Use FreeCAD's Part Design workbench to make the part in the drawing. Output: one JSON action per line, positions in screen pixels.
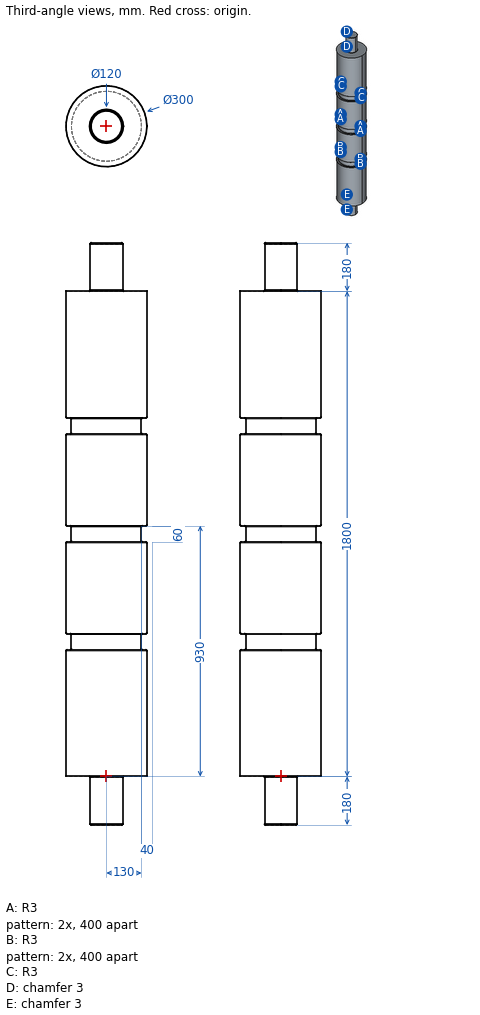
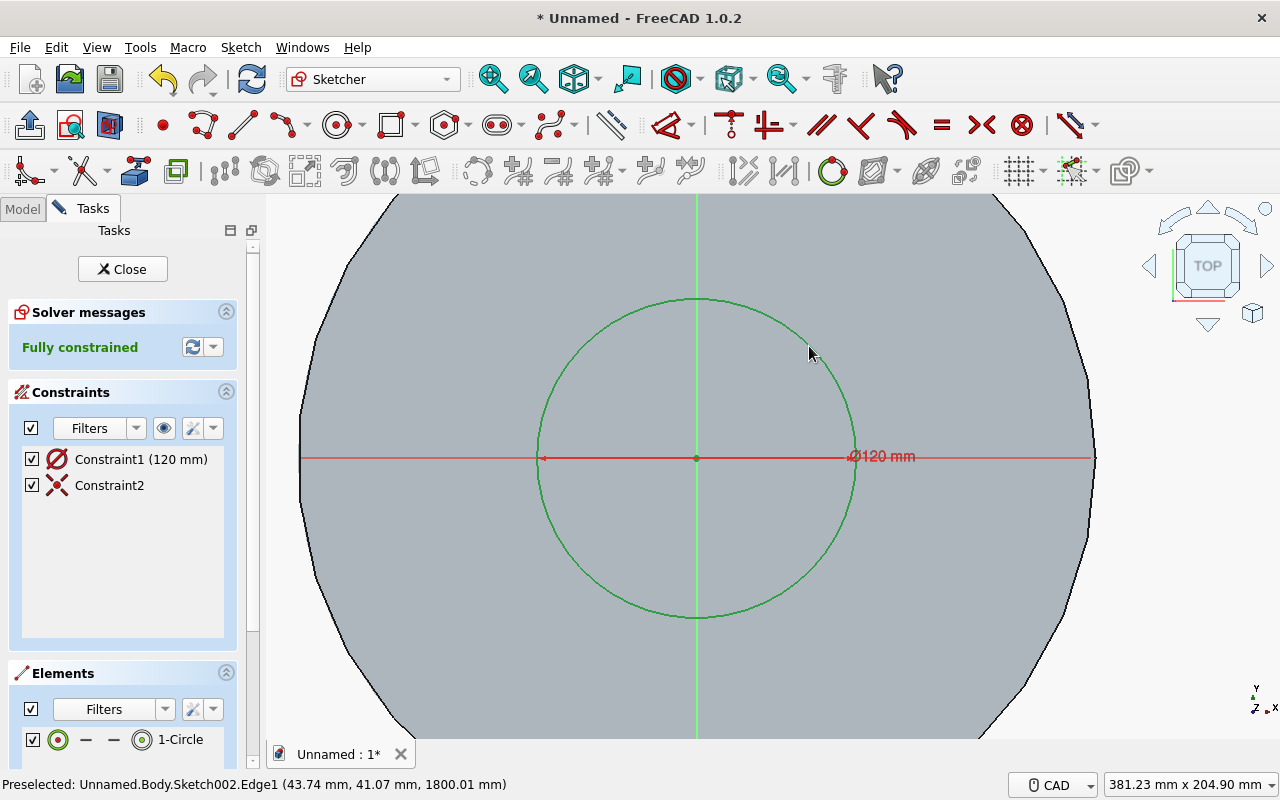
{"action": "left_click", "coordinate": [123, 269]}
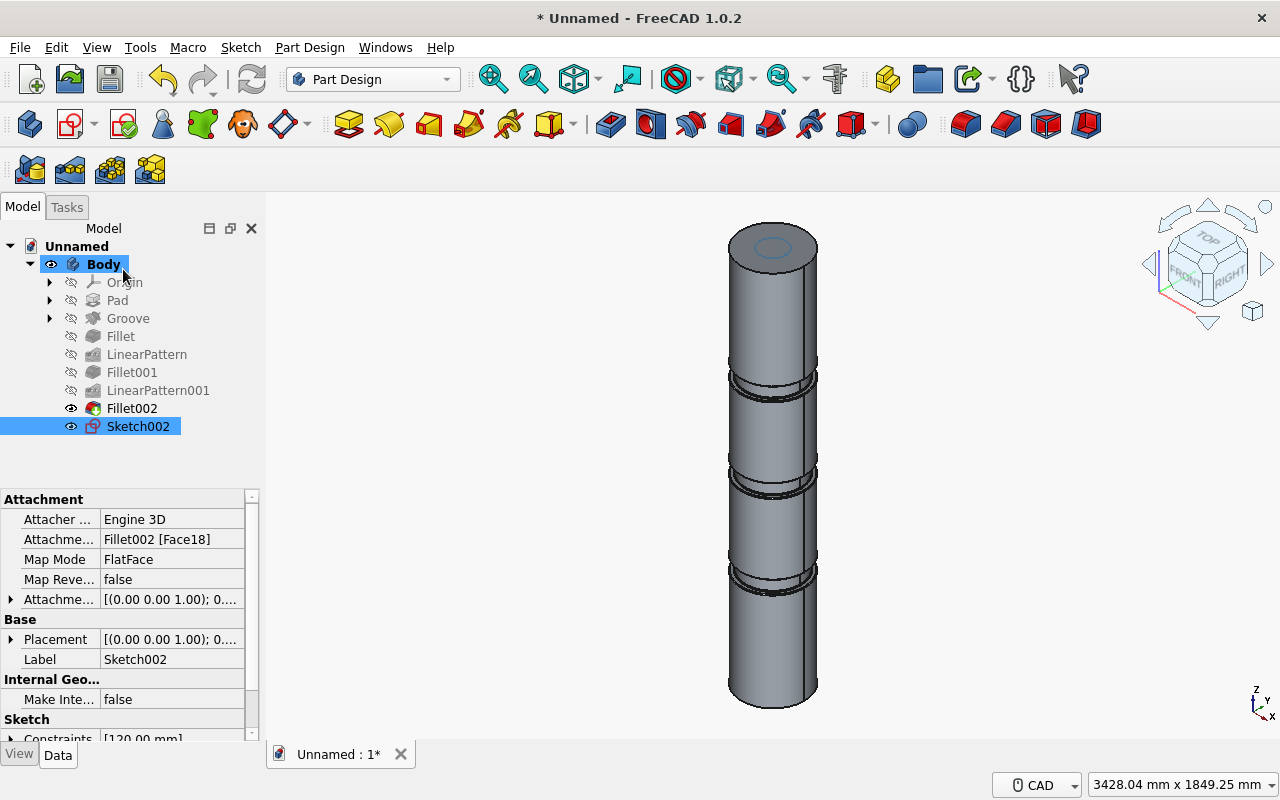
{"action": "left_click", "coordinate": [350, 124]}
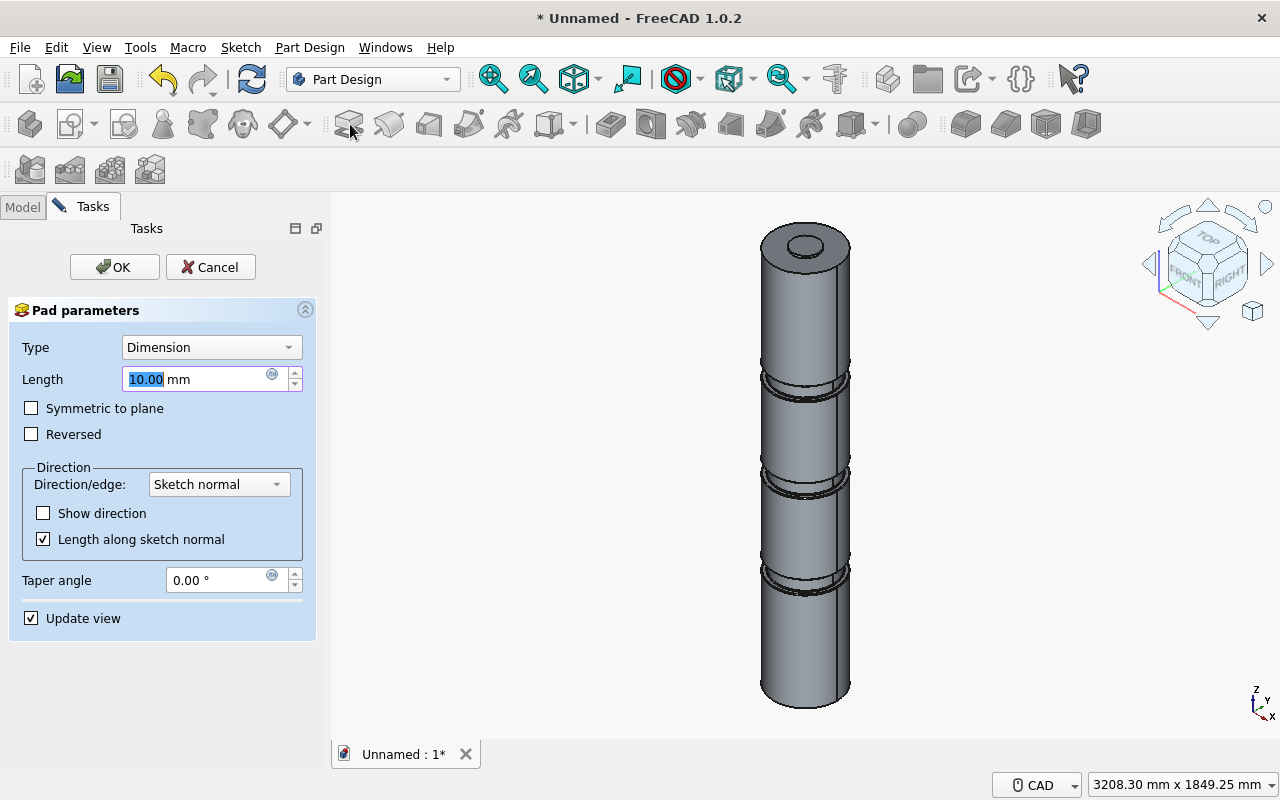
{"action": "type", "text": "180"}
{"action": "key", "text": "Tab"}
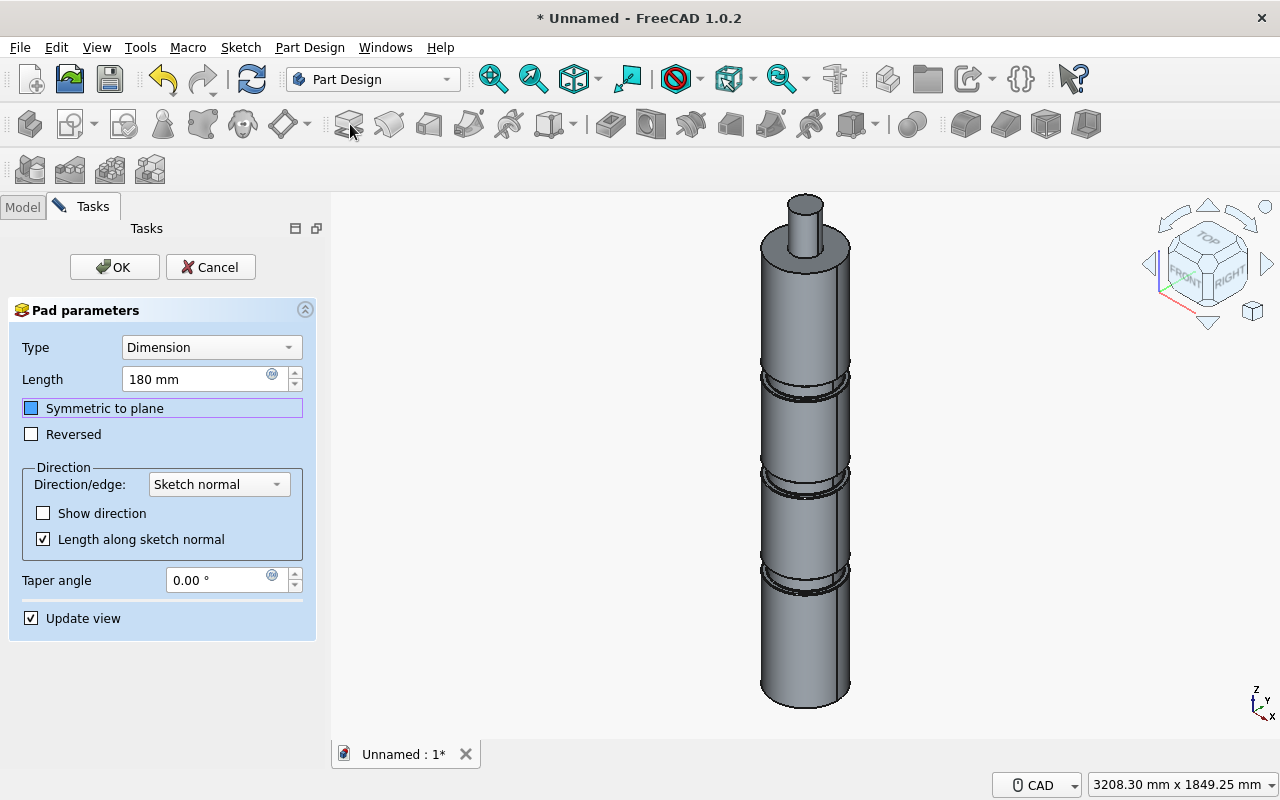
{"action": "left_click", "coordinate": [115, 267]}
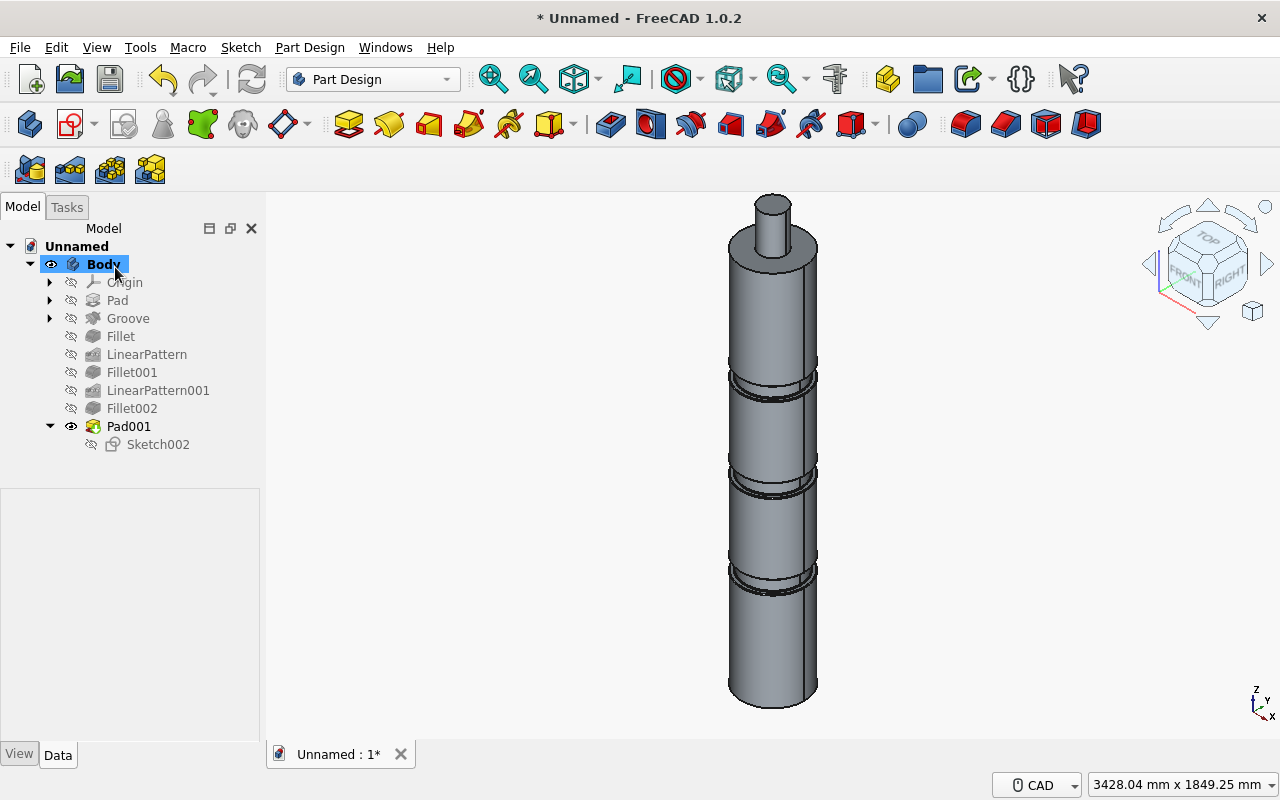
{"action": "left_click", "coordinate": [494, 80]}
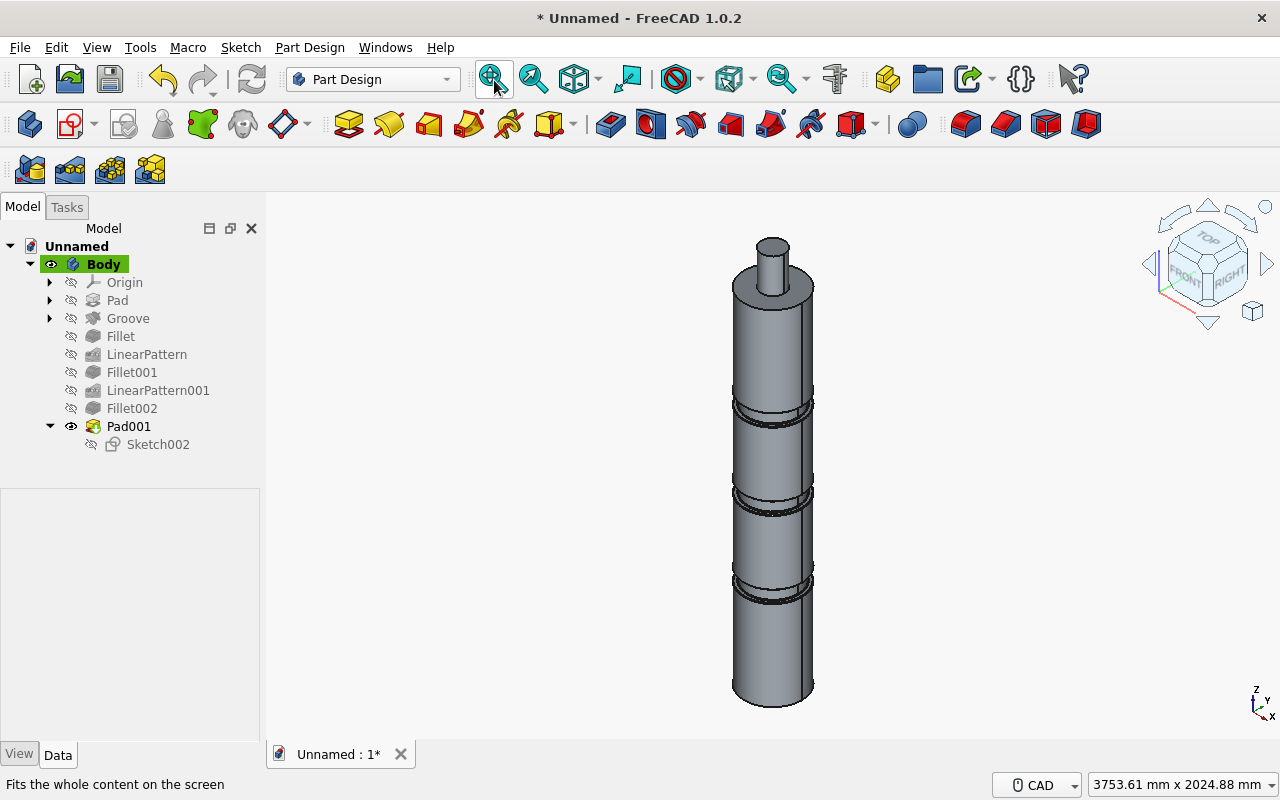
{"action": "left_click", "coordinate": [762, 240]}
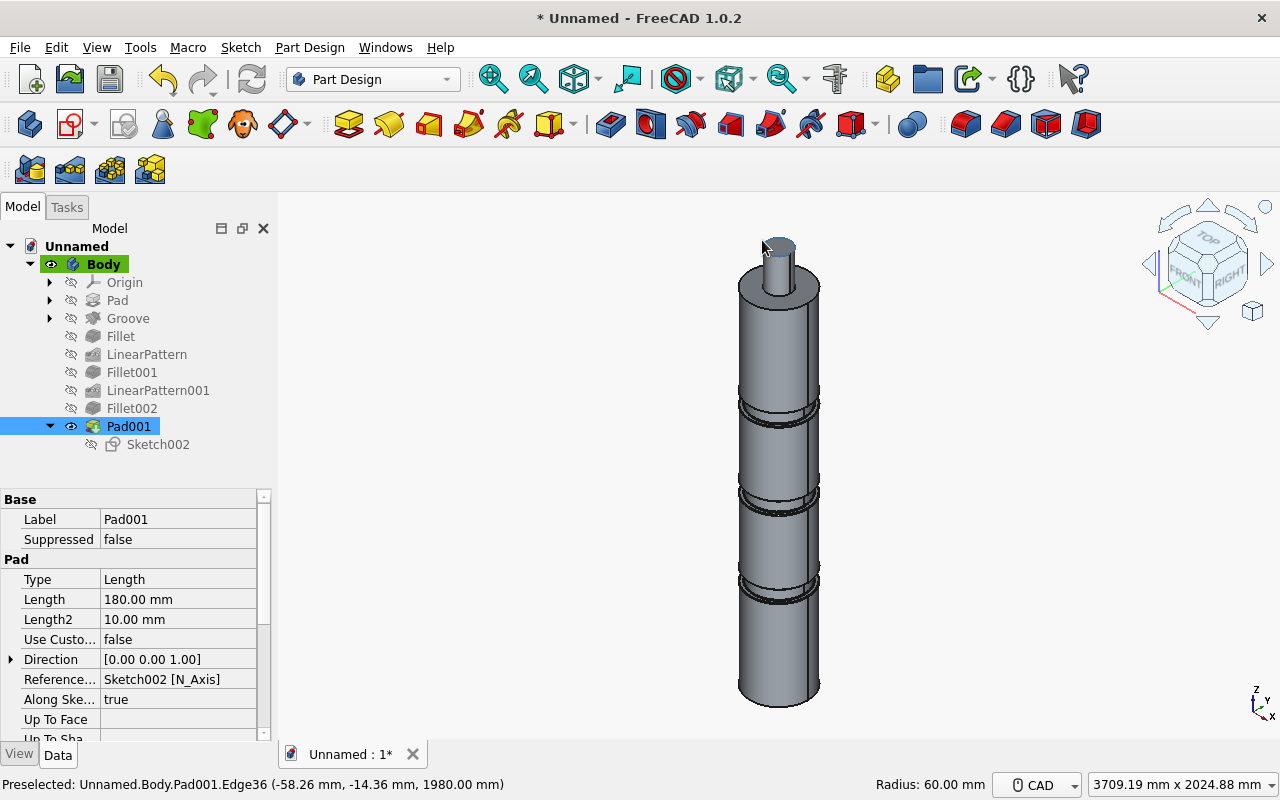
{"action": "key", "text": "2"}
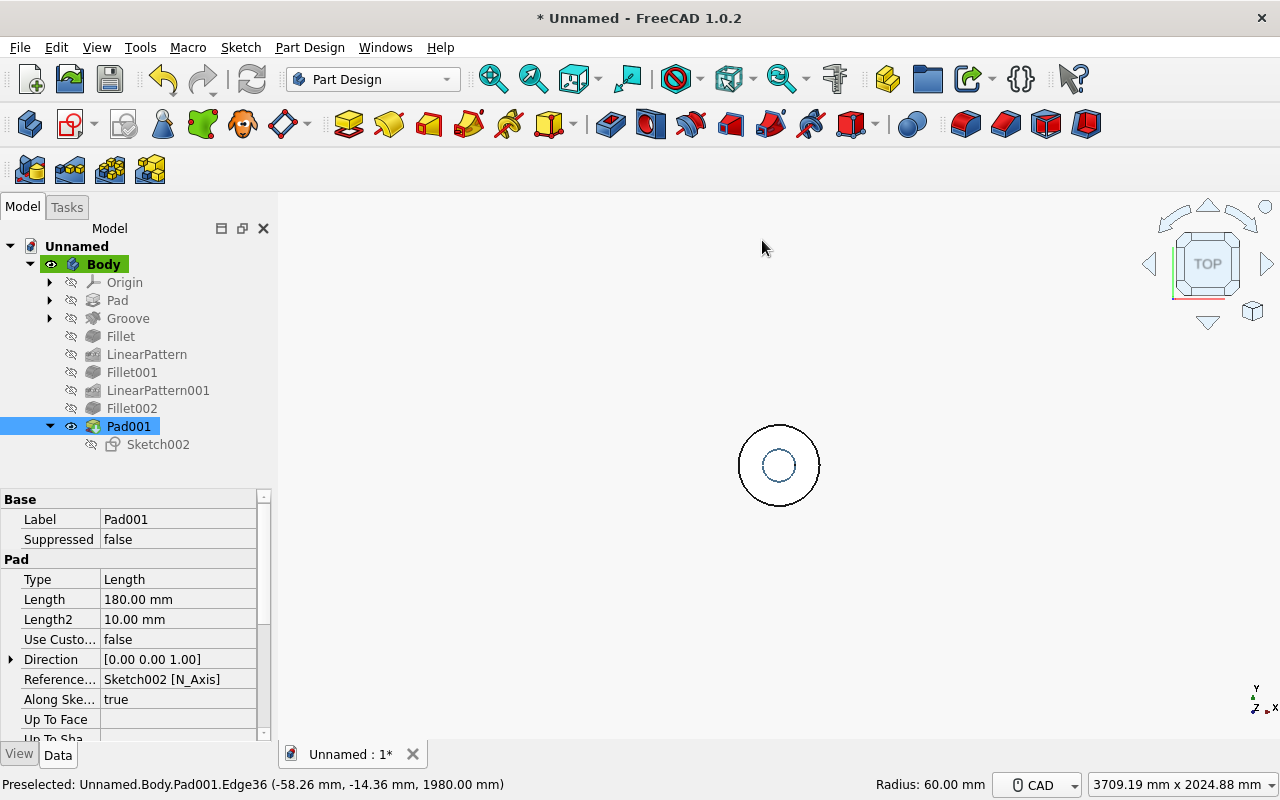
{"action": "left_click", "coordinate": [494, 80]}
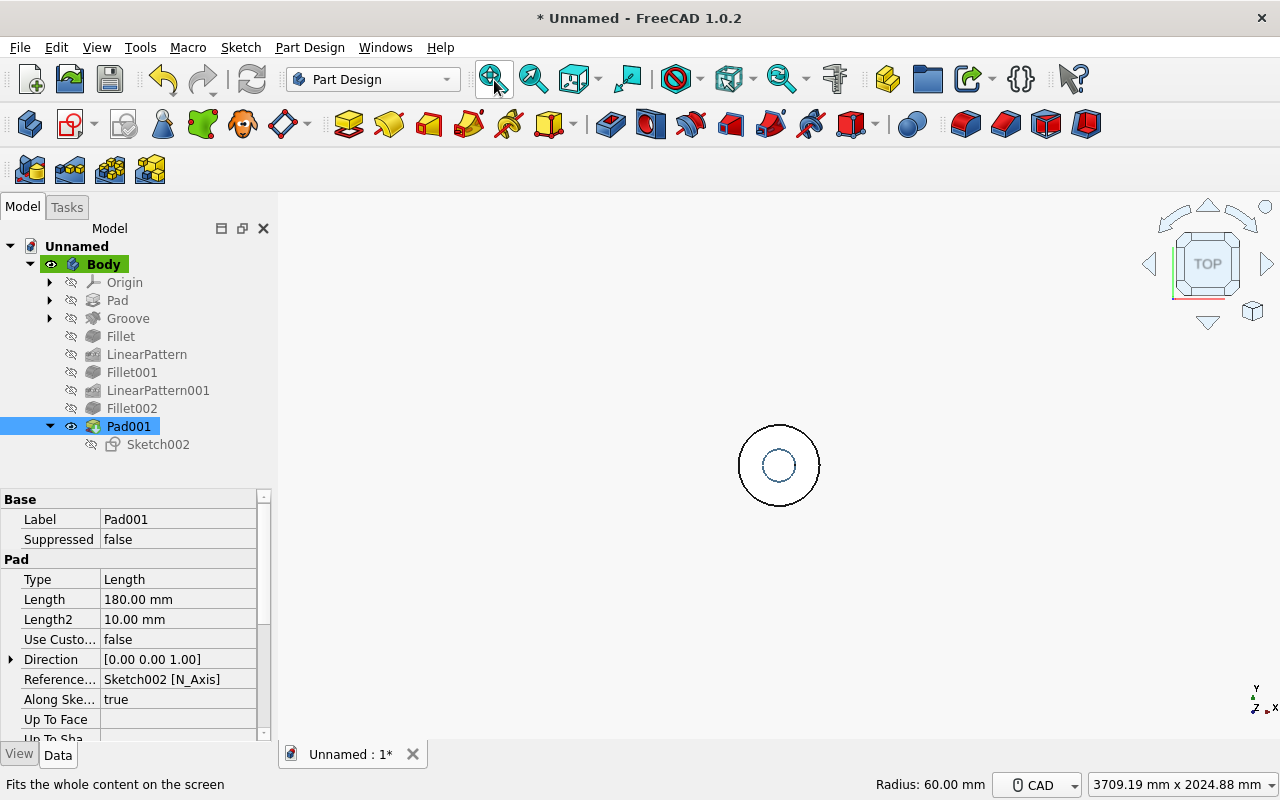
{"action": "key", "text": "0"}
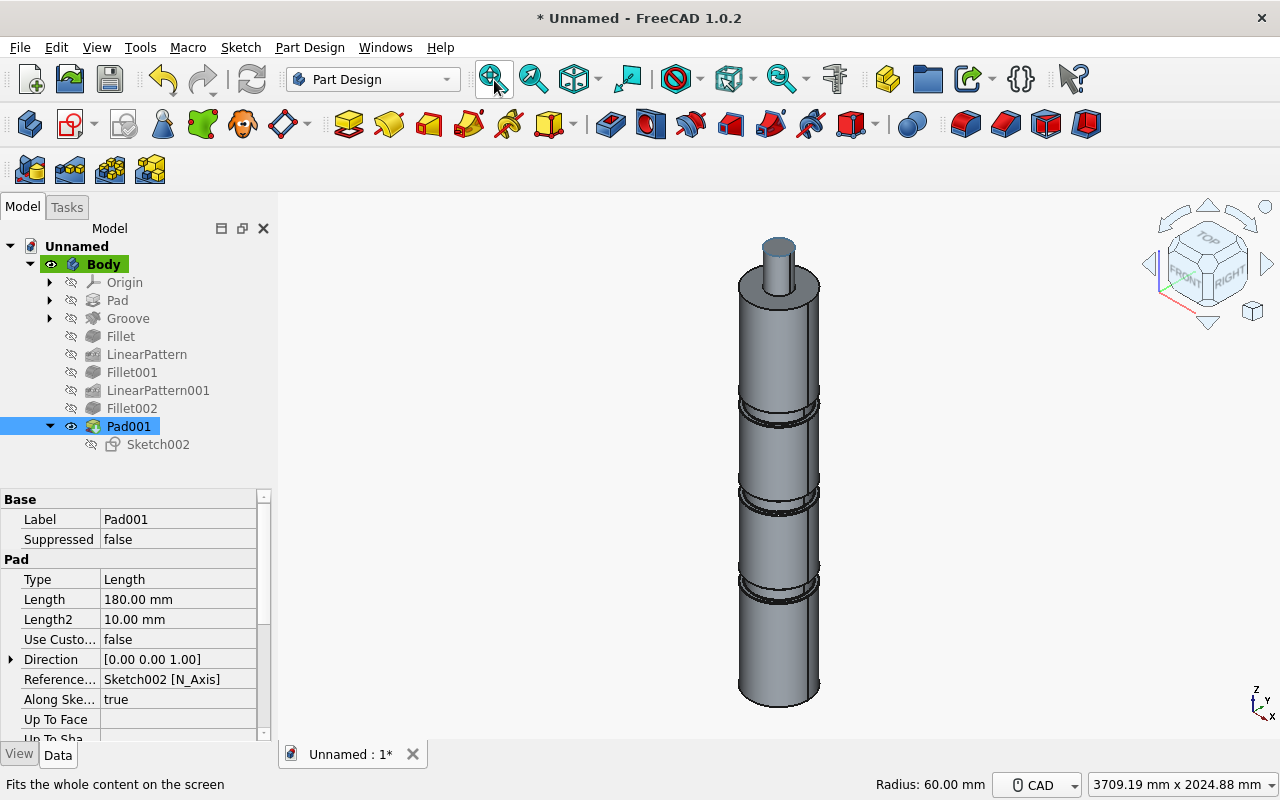
{"action": "key", "text": "1"}